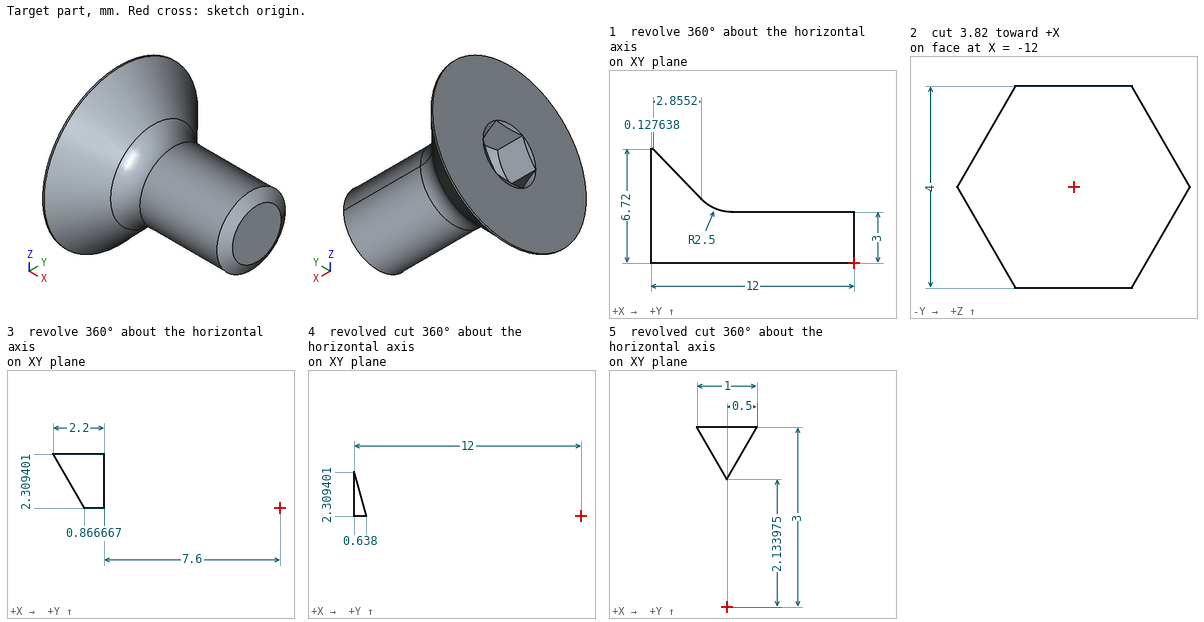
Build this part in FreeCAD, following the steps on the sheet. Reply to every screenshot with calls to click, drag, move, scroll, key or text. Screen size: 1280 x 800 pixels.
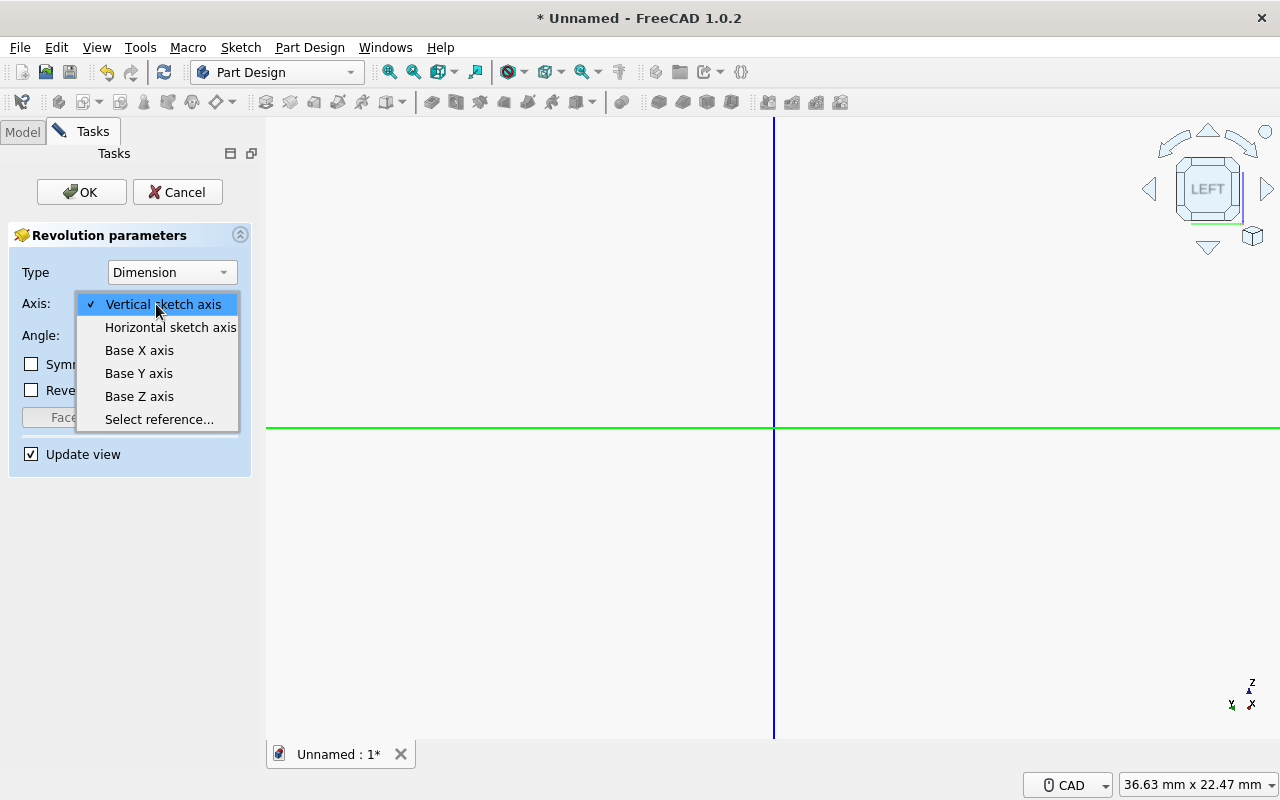
click(156, 328)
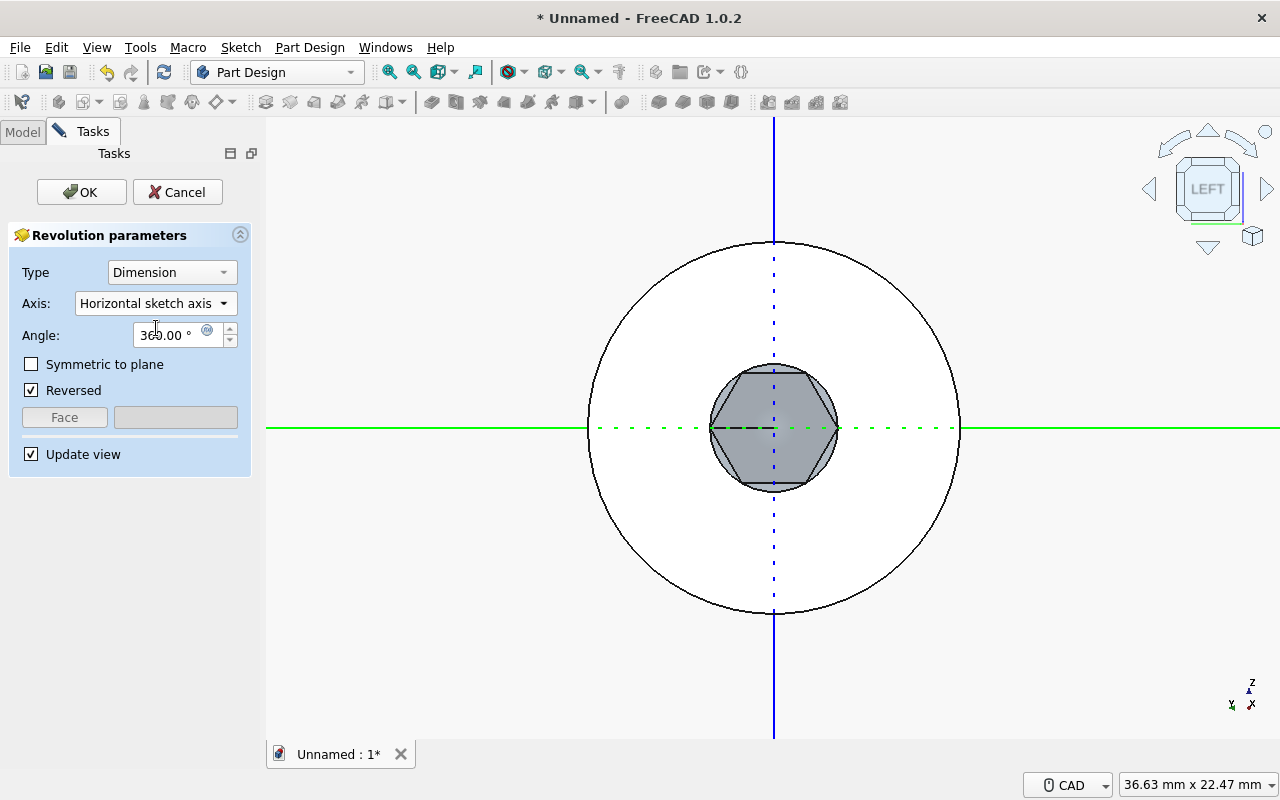
click(82, 192)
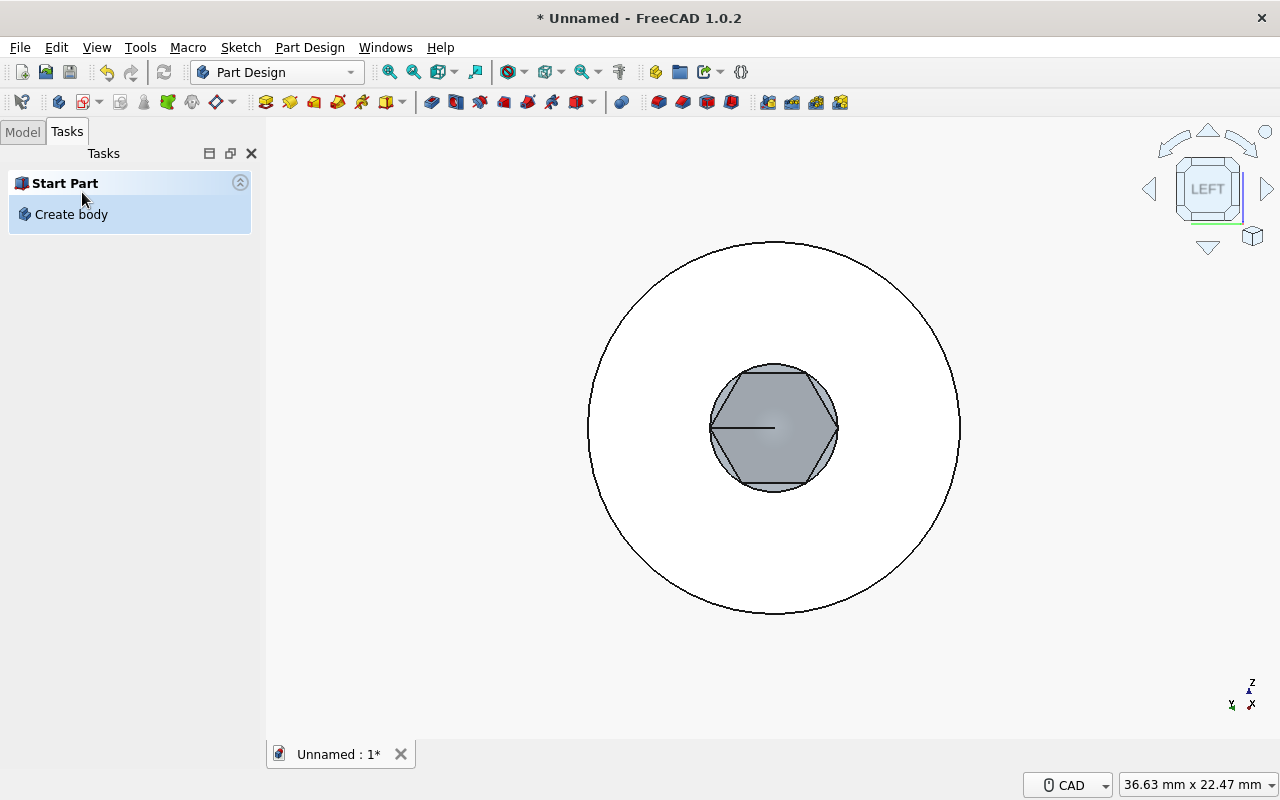
key(0)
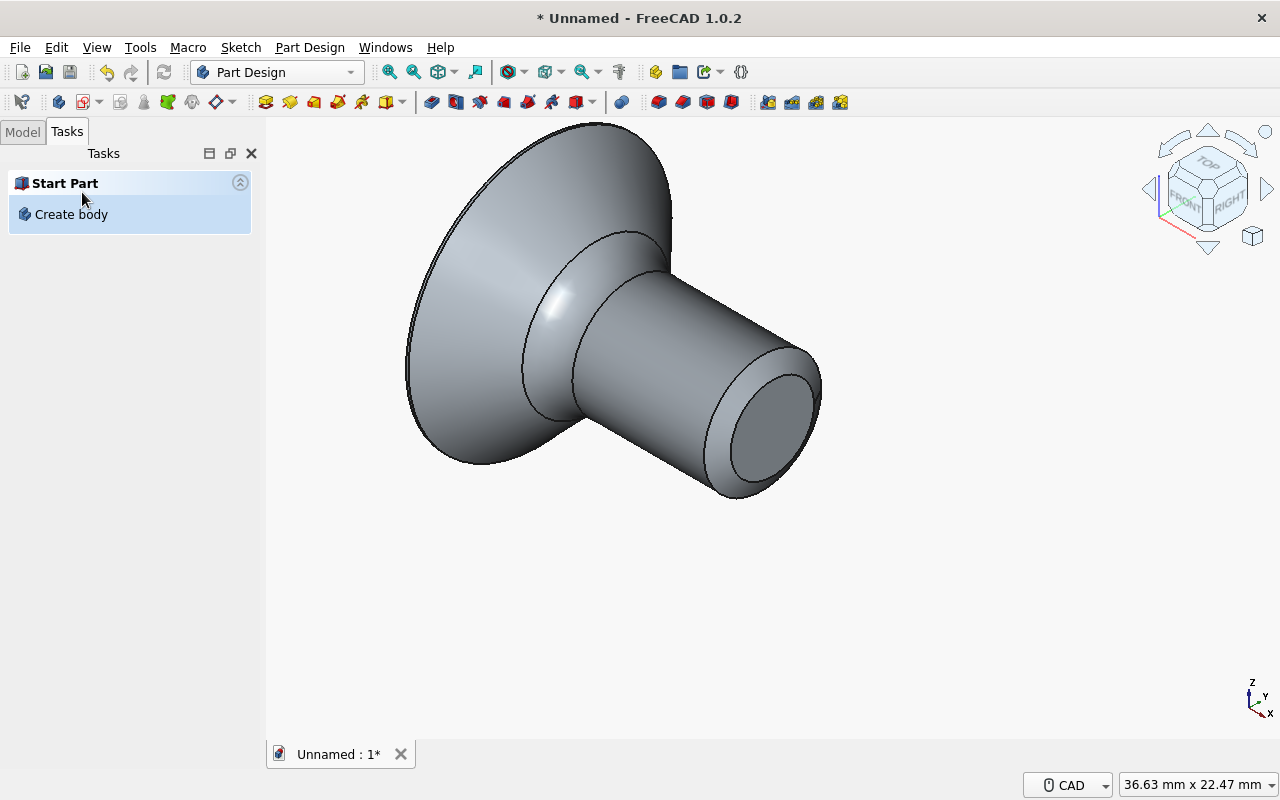
key(v)
key(f)